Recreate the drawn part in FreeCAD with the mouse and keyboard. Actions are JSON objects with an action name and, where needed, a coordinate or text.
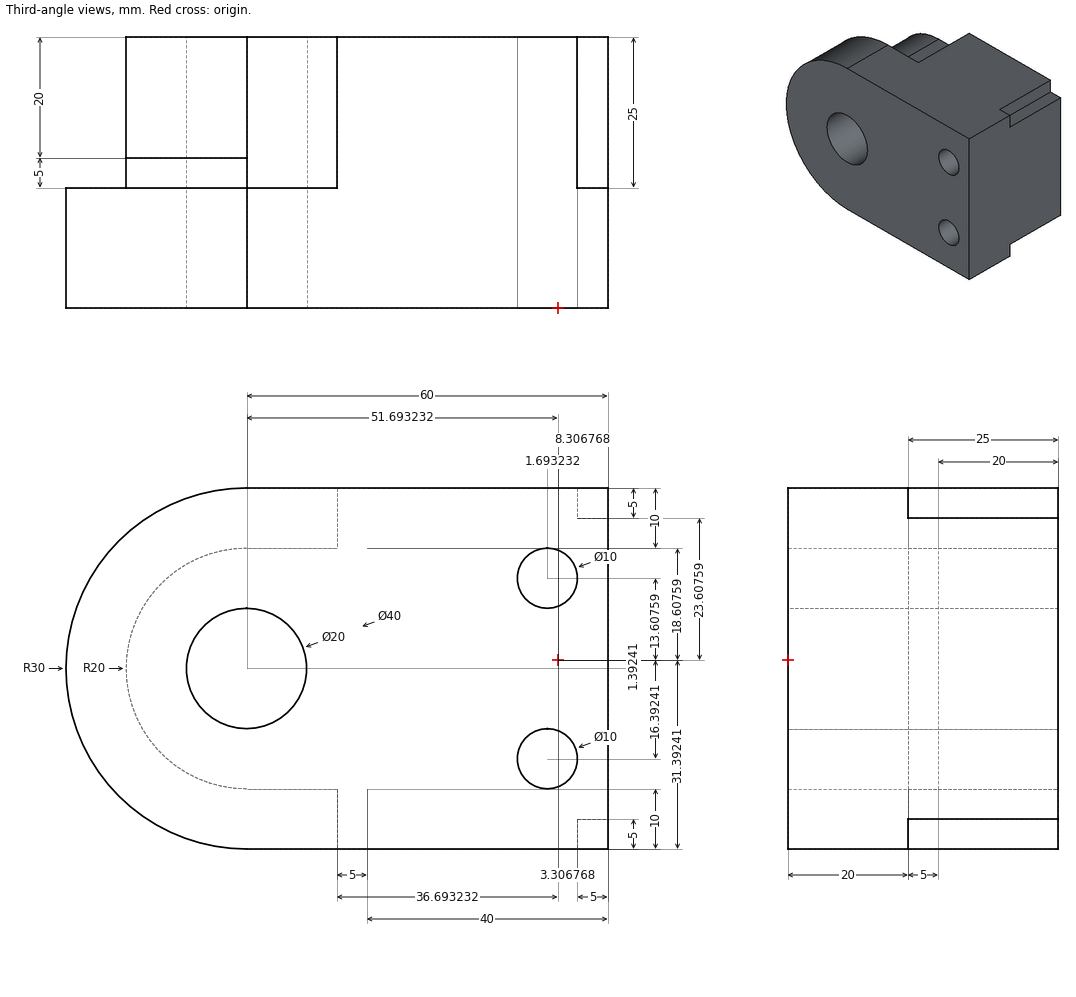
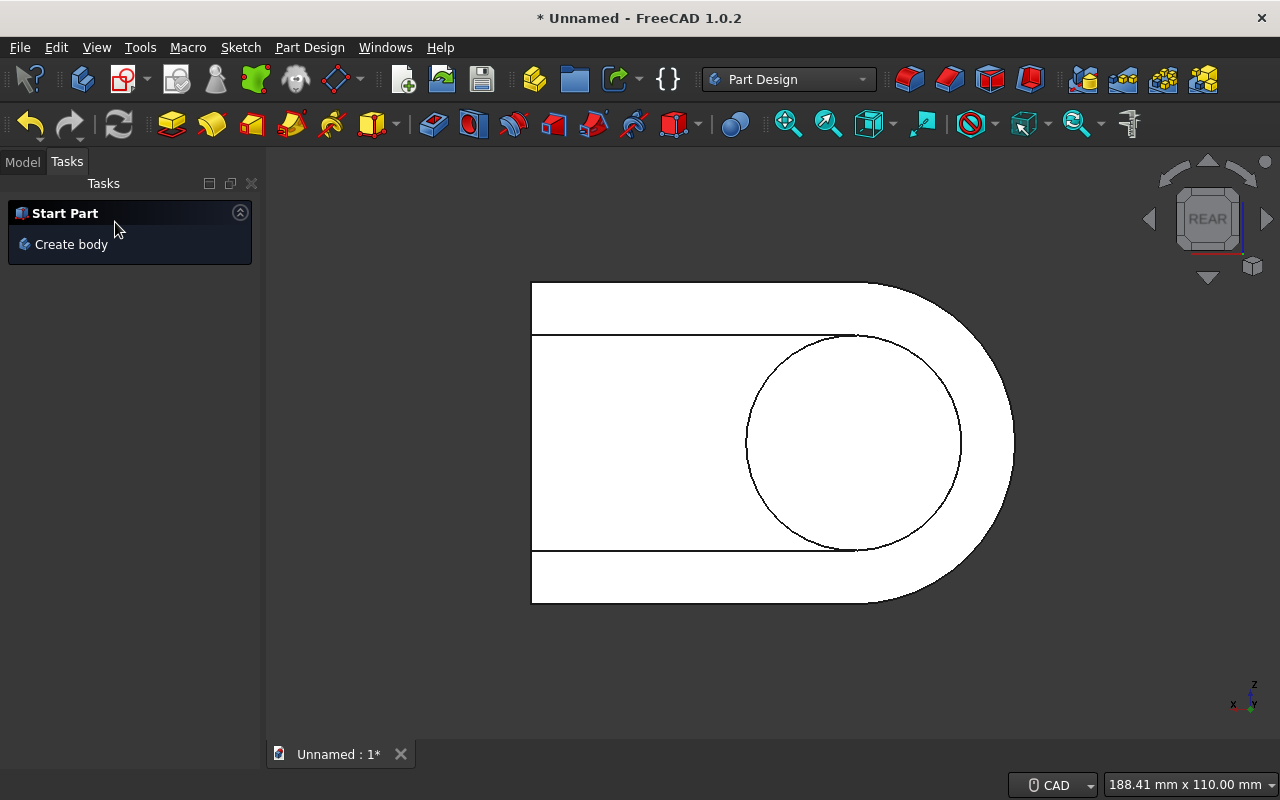
{"action": "left_click", "coordinate": [646, 442]}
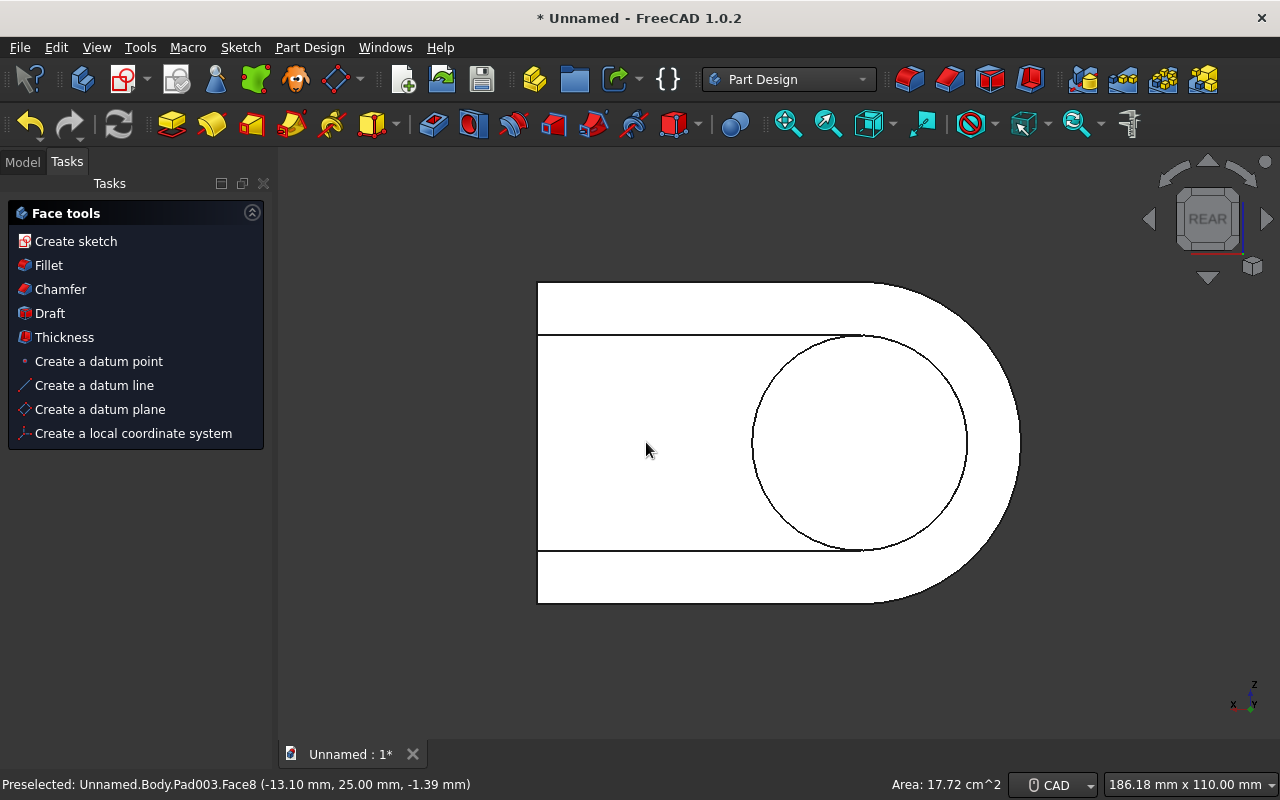
{"action": "left_click", "coordinate": [124, 80]}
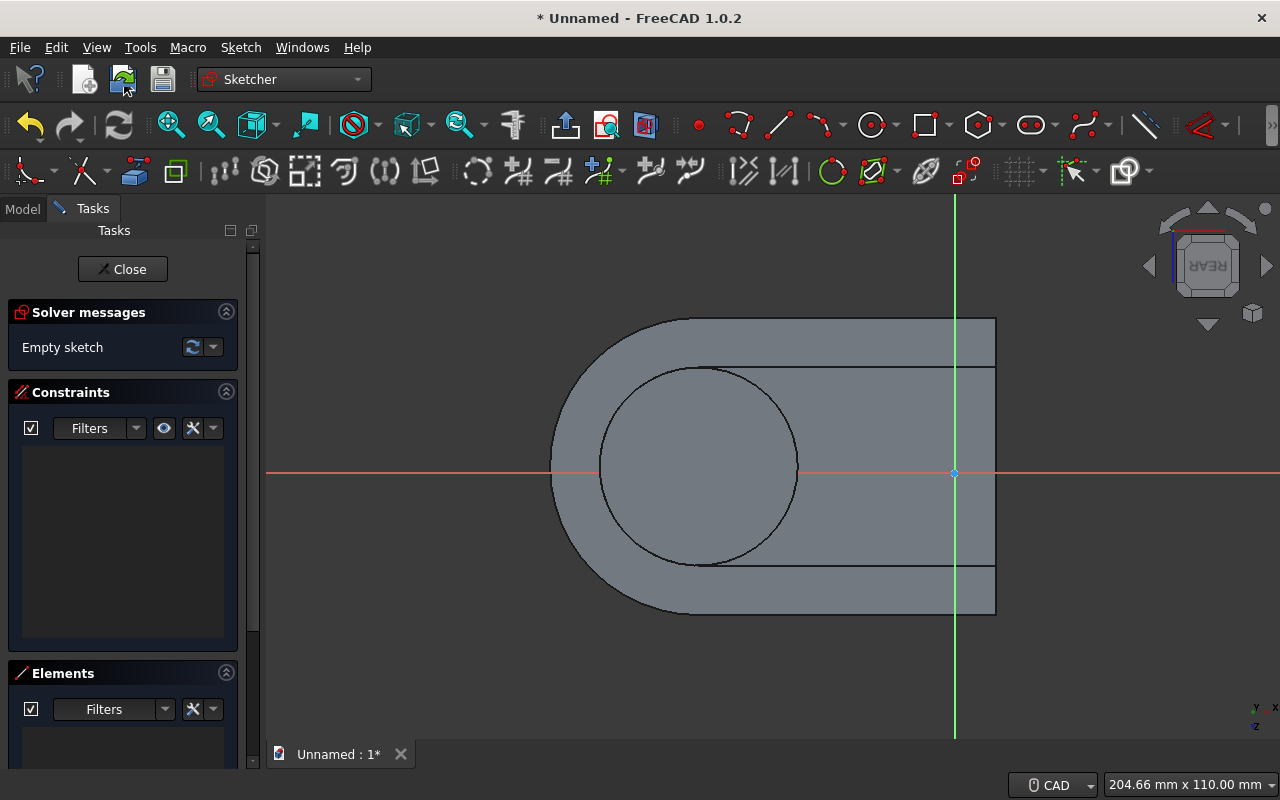
{"action": "key", "text": "q s"}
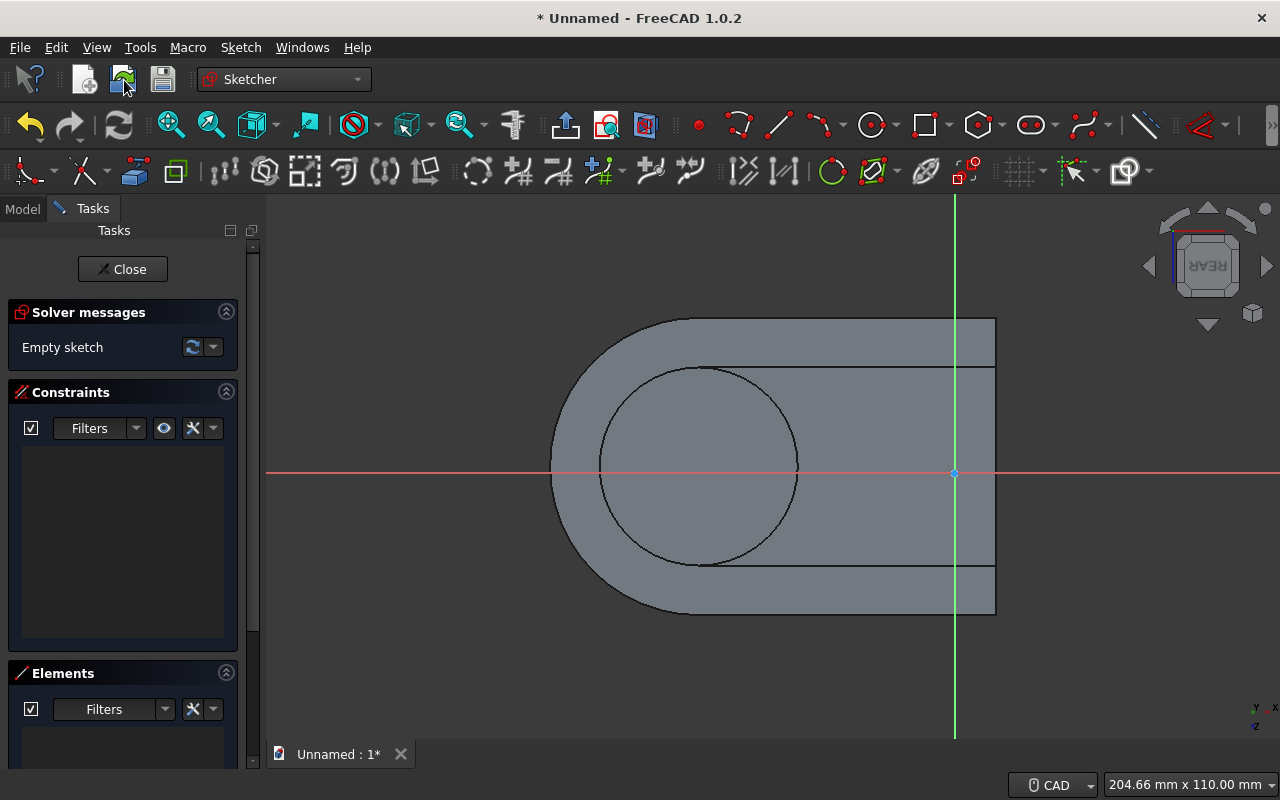
{"action": "scroll", "coordinate": [1021, 466], "scroll_direction": "up", "scroll_amount": 3}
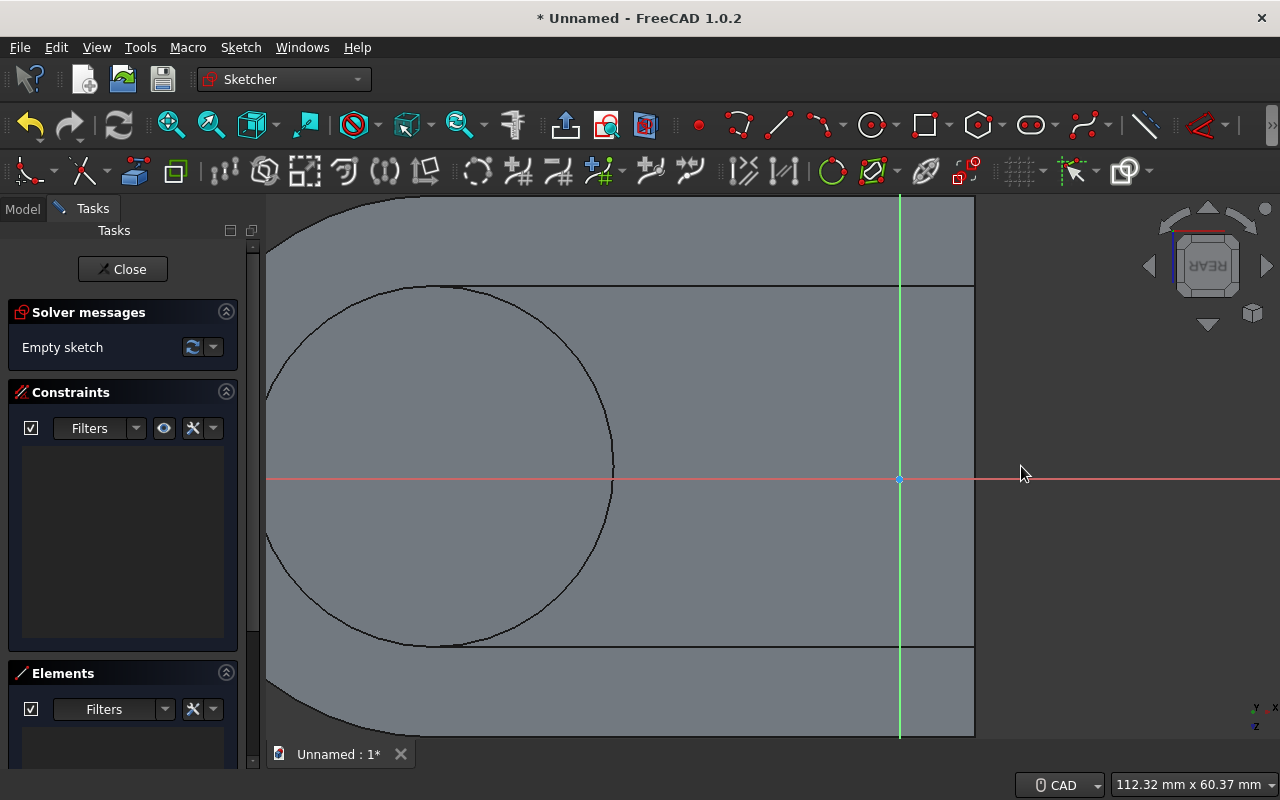
{"action": "key", "text": "g m"}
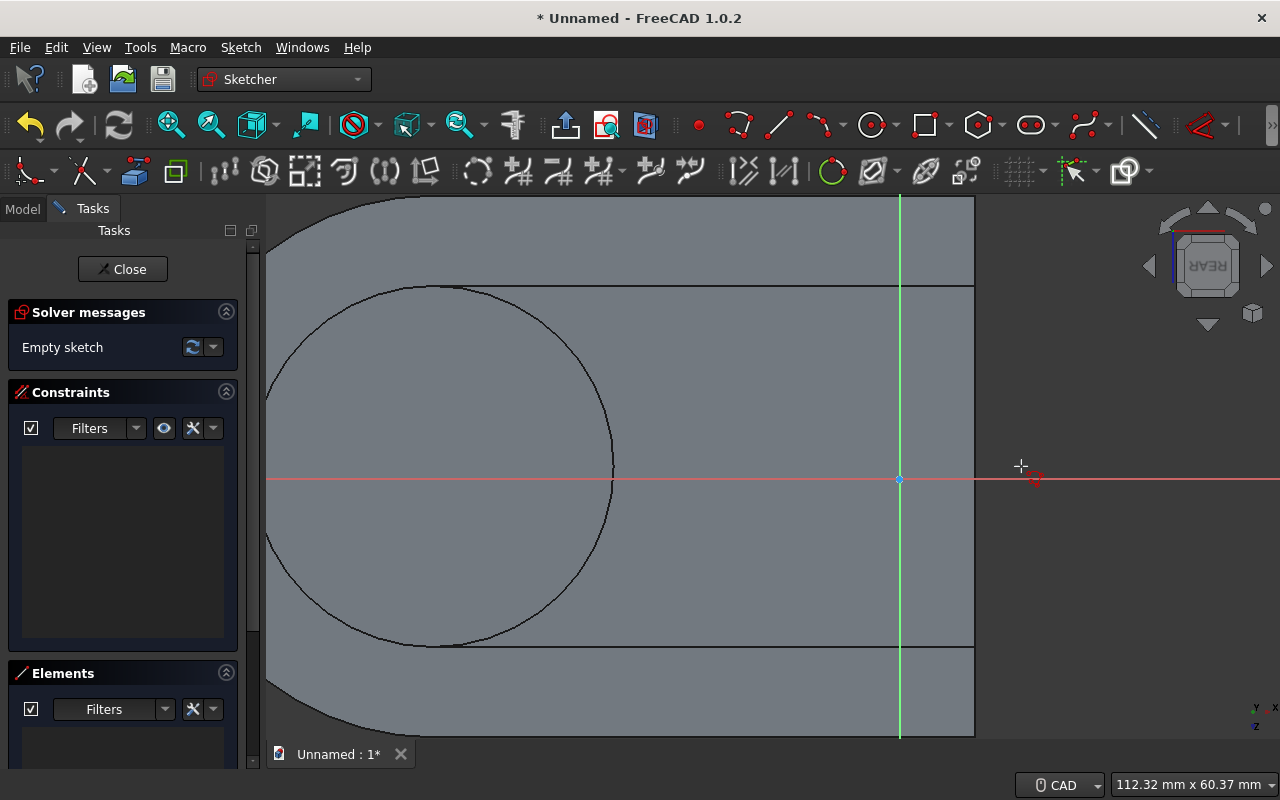
{"action": "left_click", "coordinate": [433, 647]}
{"action": "left_click", "coordinate": [975, 647]}
{"action": "left_click", "coordinate": [975, 286]}
{"action": "left_click", "coordinate": [433, 286]}
{"action": "right_click", "coordinate": [433, 286]}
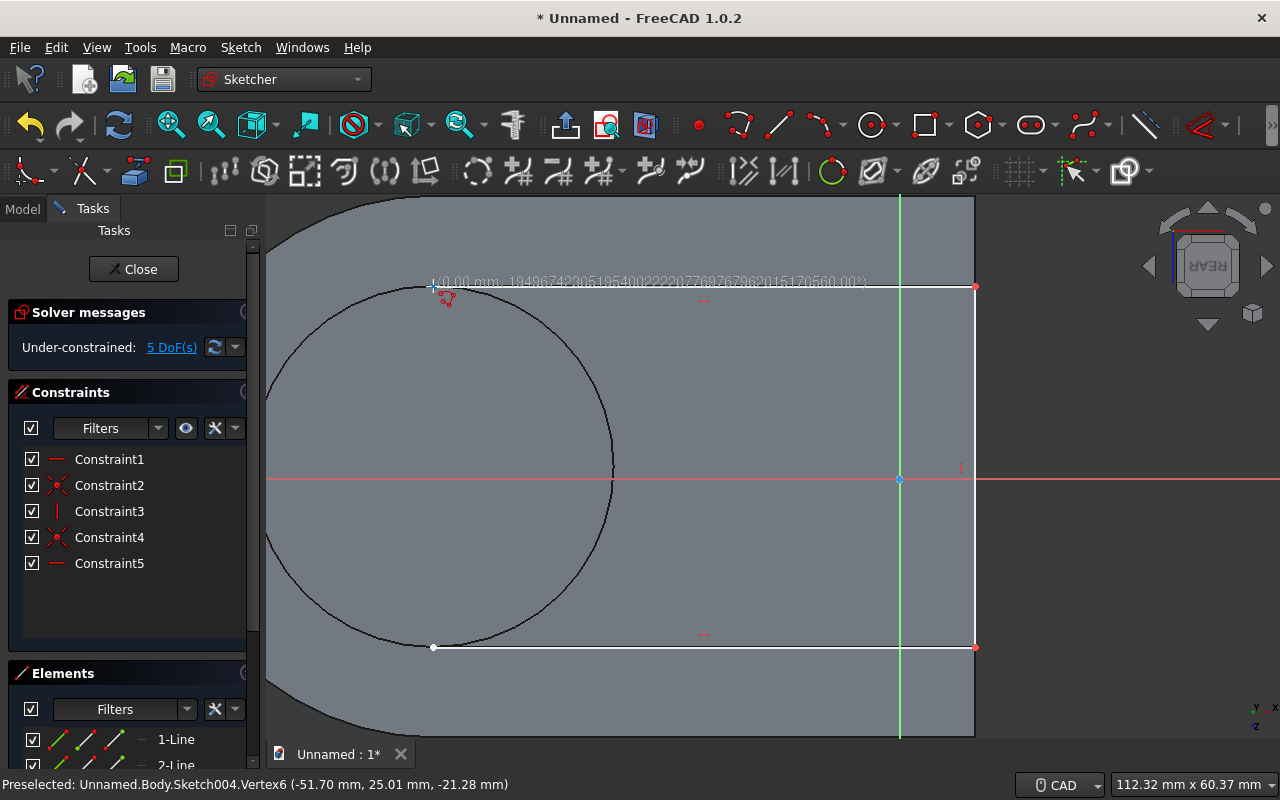
{"action": "left_click", "coordinate": [820, 126]}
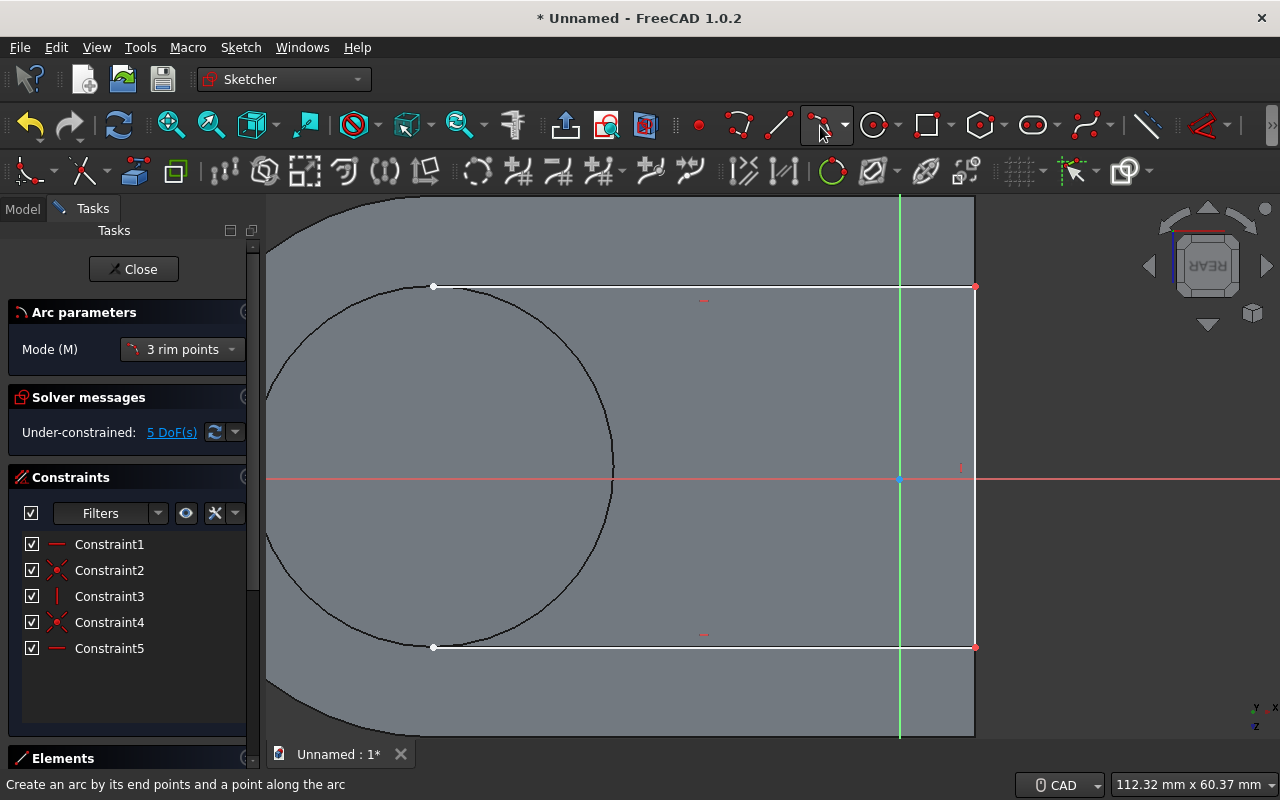
{"action": "left_click", "coordinate": [433, 287]}
{"action": "left_click", "coordinate": [433, 648]}
{"action": "left_click", "coordinate": [605, 522]}
{"action": "key", "text": "Escape"}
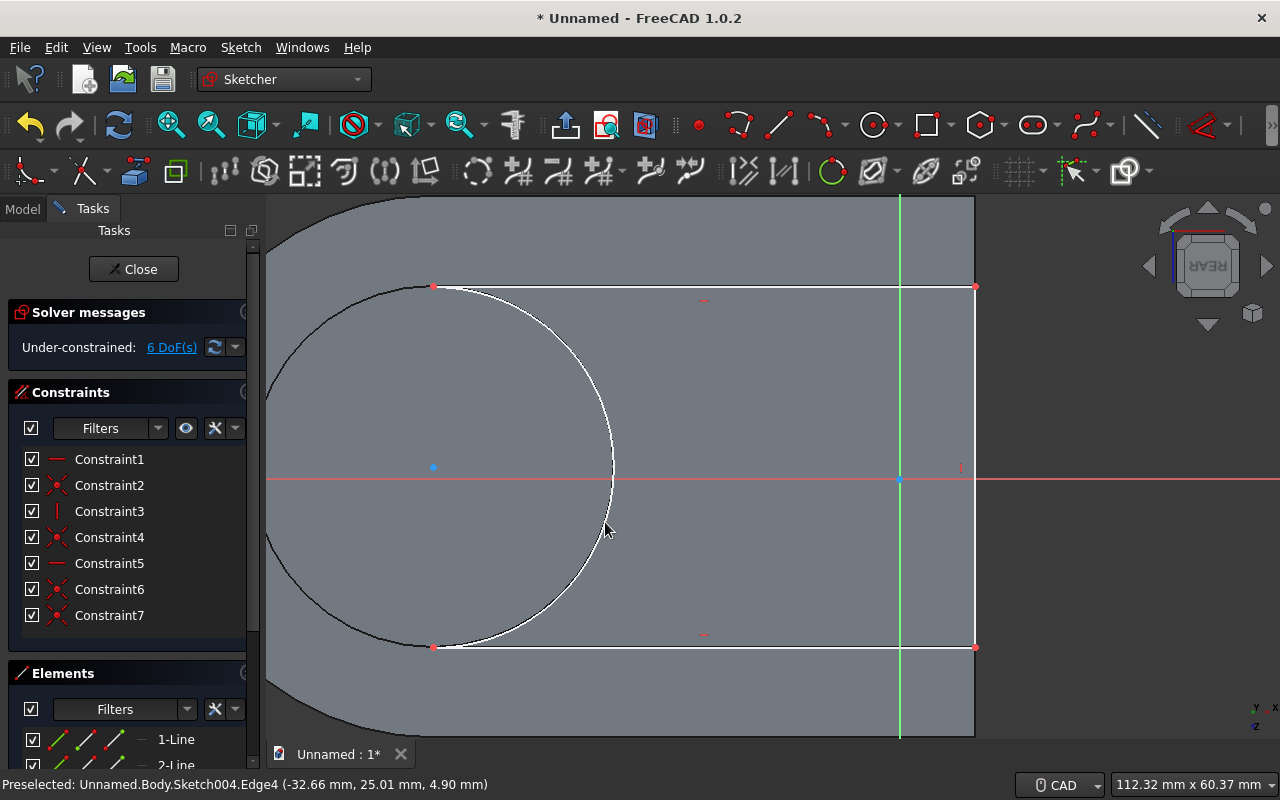
{"action": "left_click", "coordinate": [596, 648]}